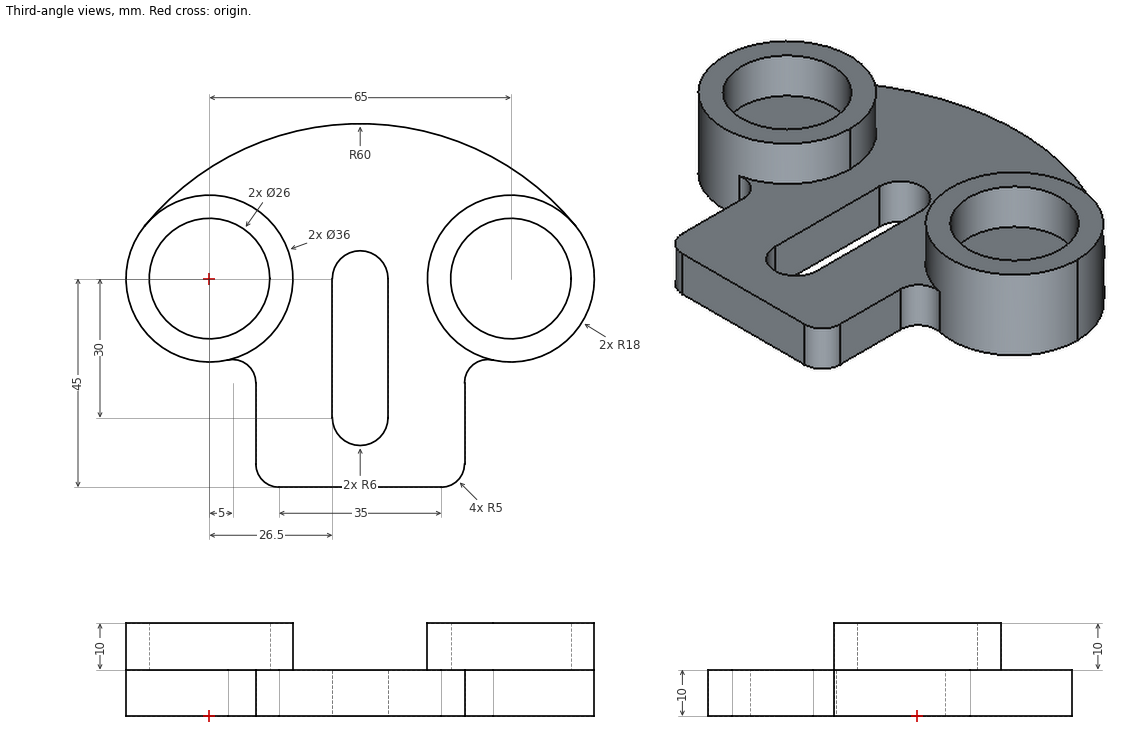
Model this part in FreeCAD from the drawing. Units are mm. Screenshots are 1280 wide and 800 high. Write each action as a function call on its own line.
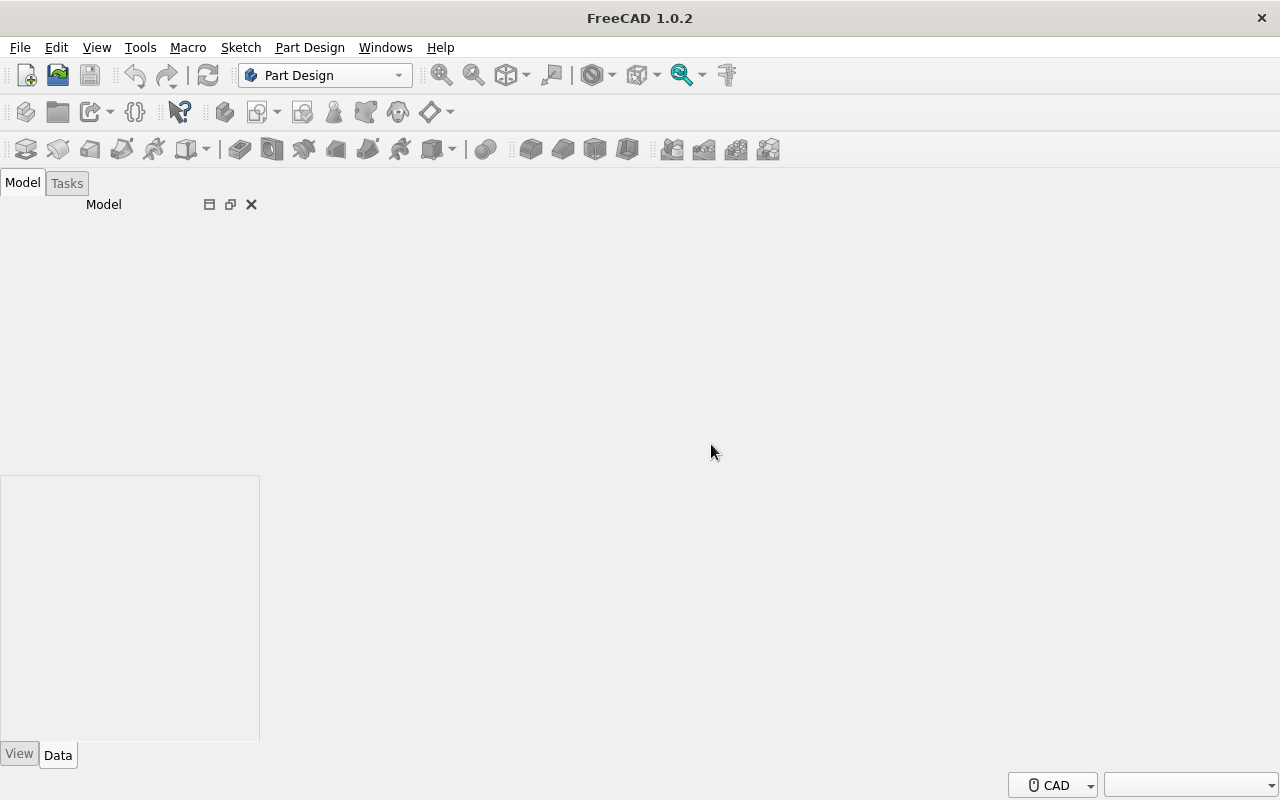
click(26, 76)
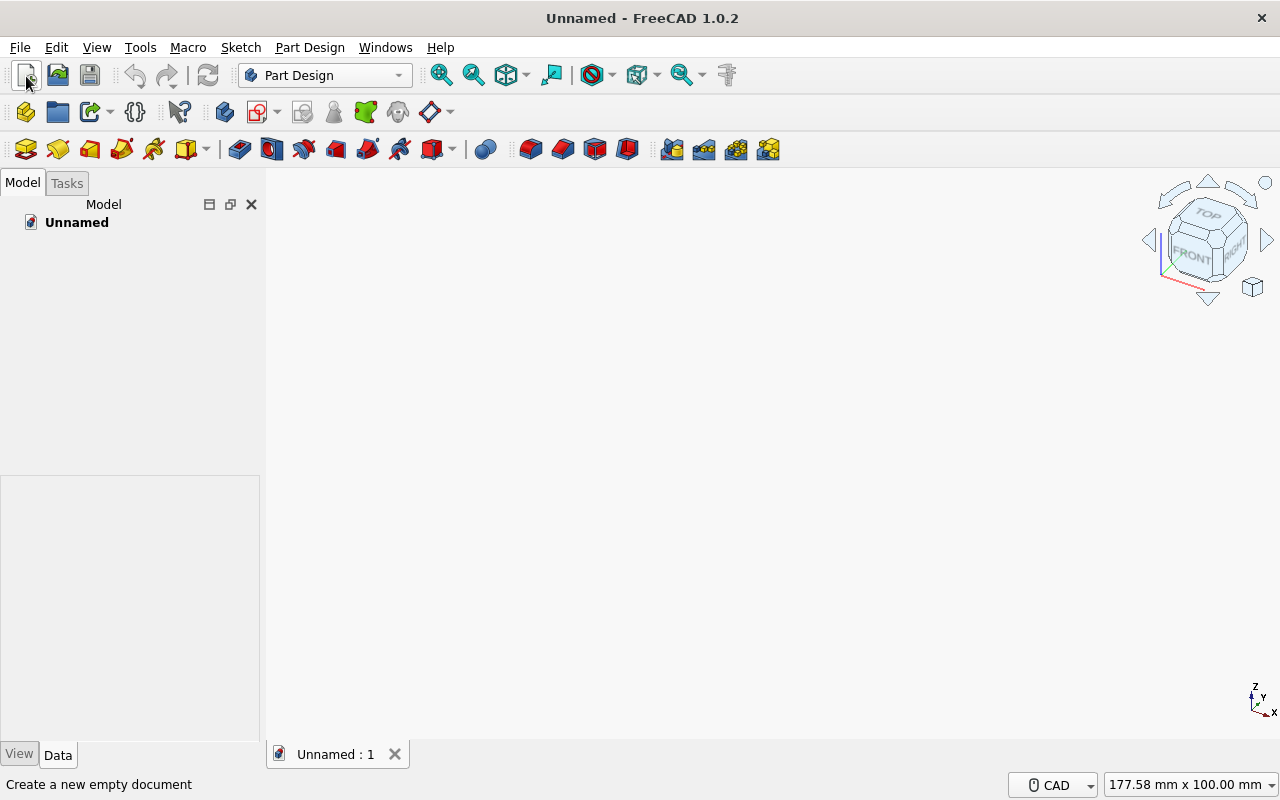
click(258, 112)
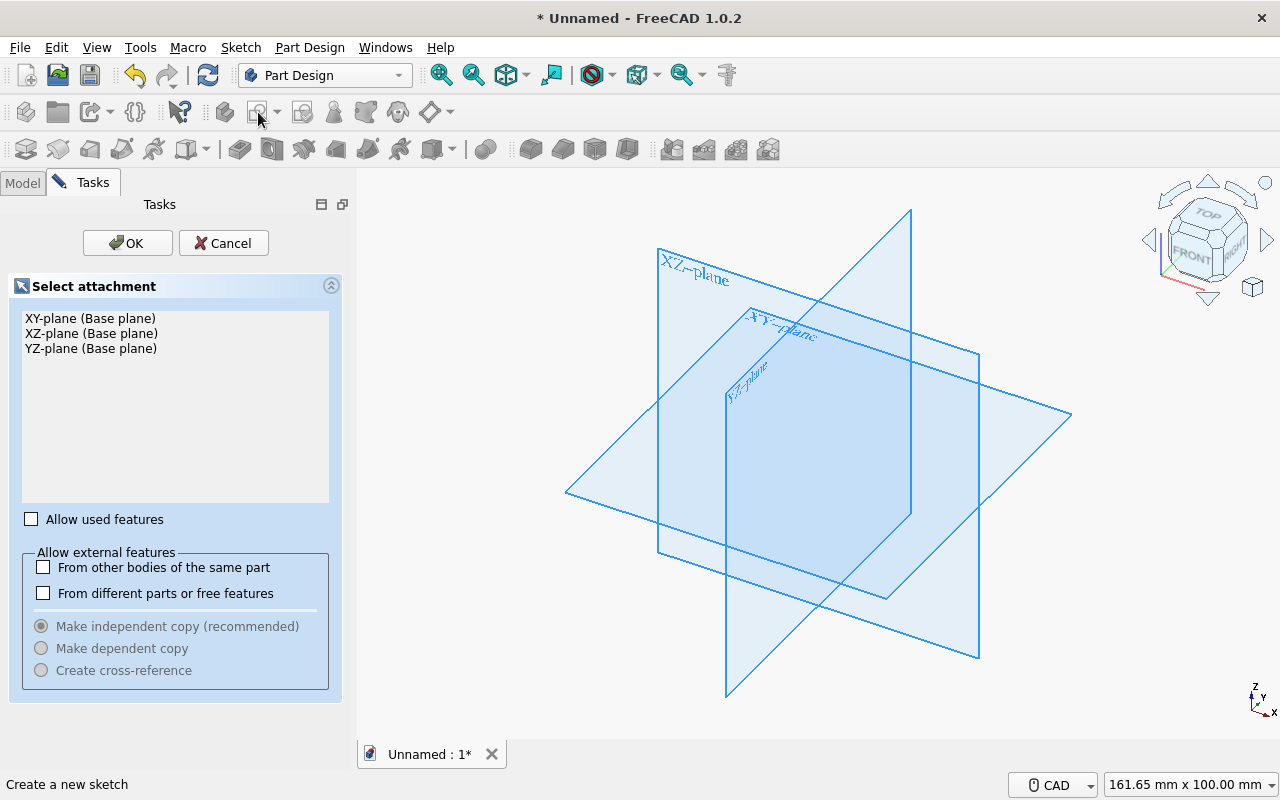
click(82, 318)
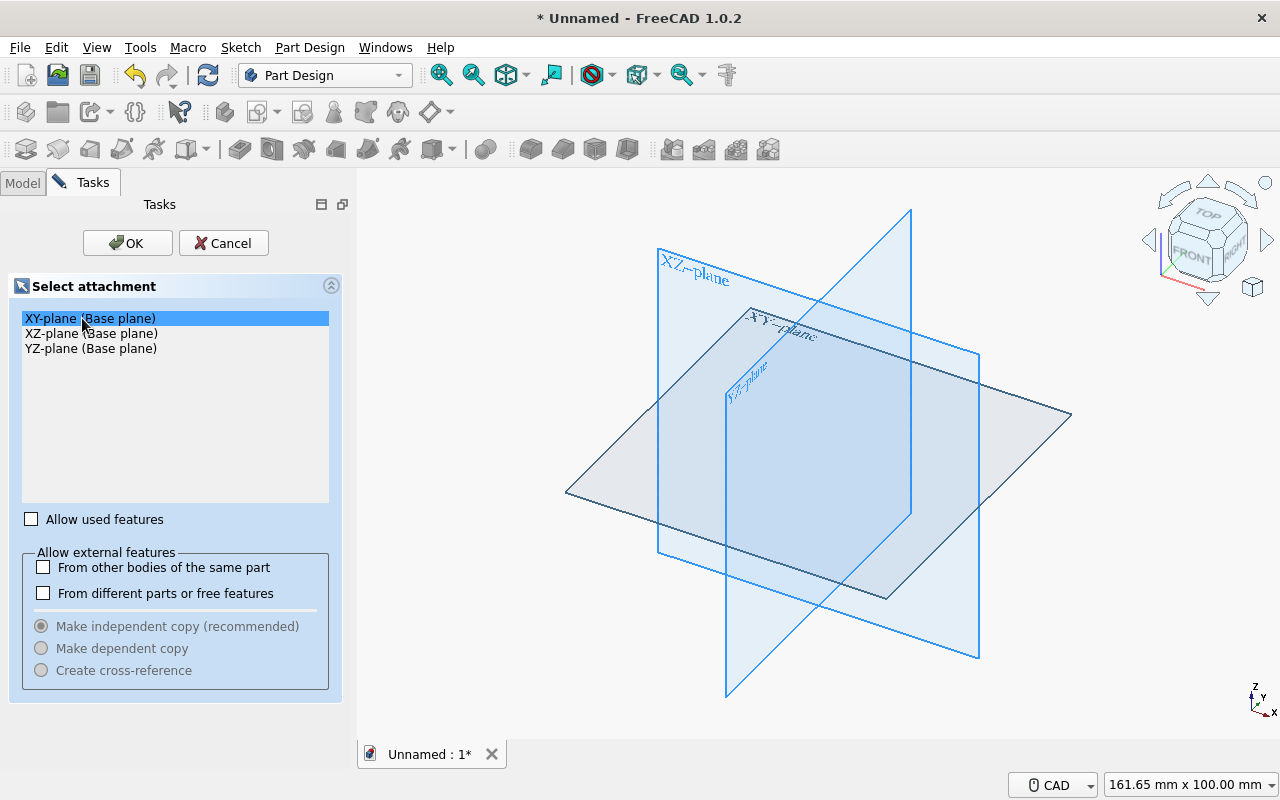
click(128, 243)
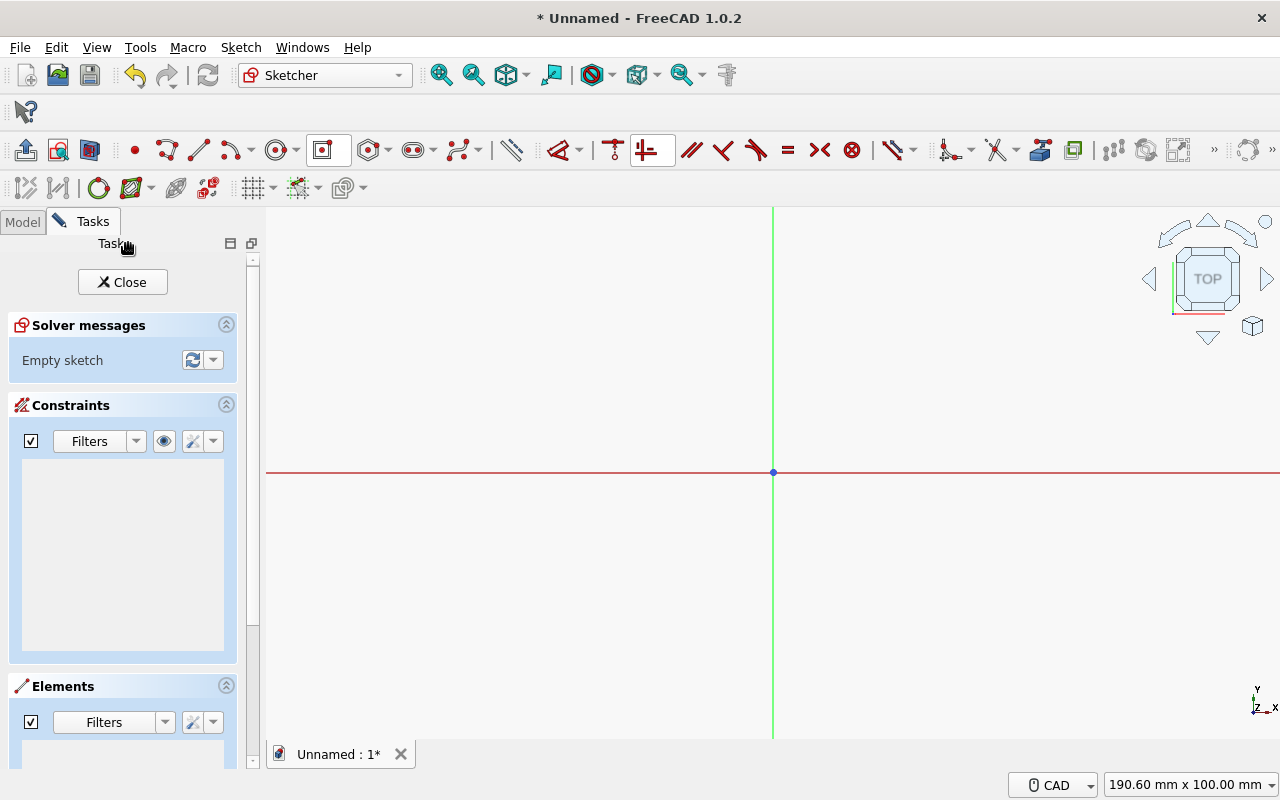
scroll(294, 334, down, 1)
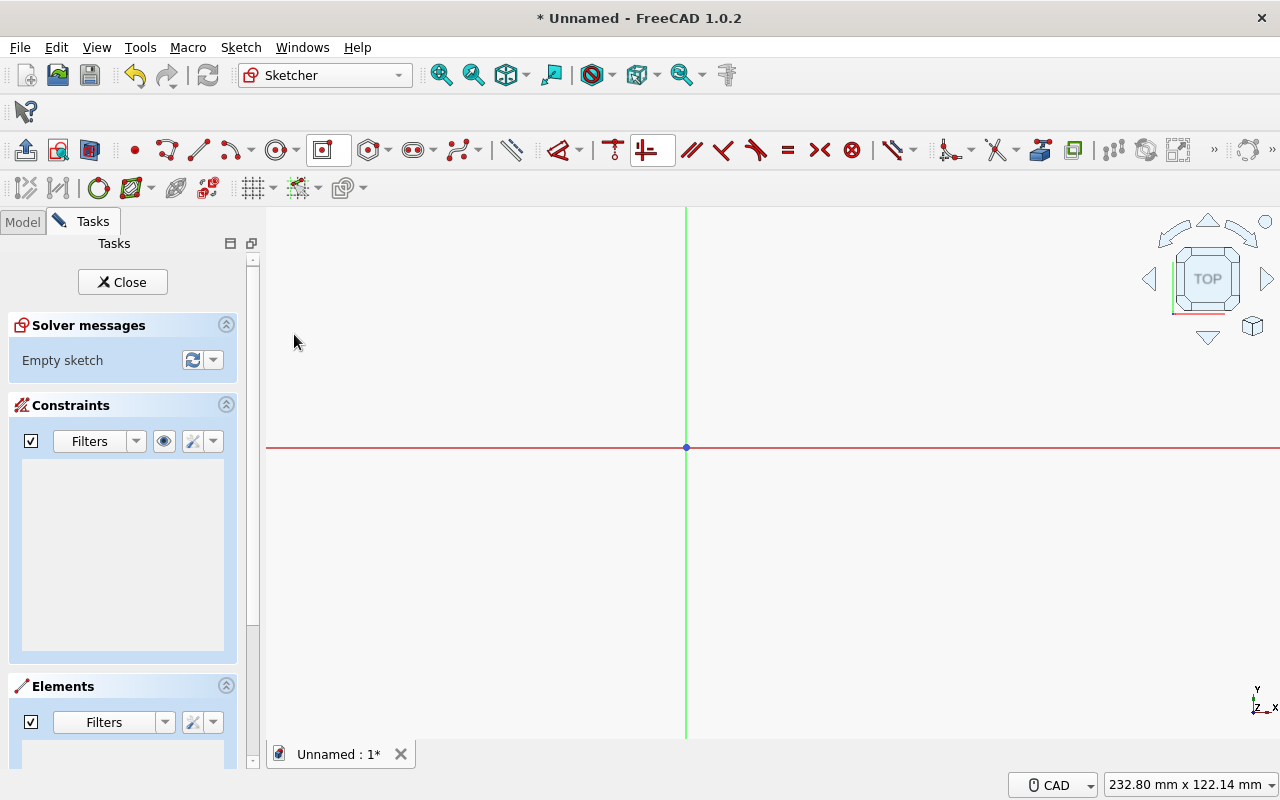
click(200, 150)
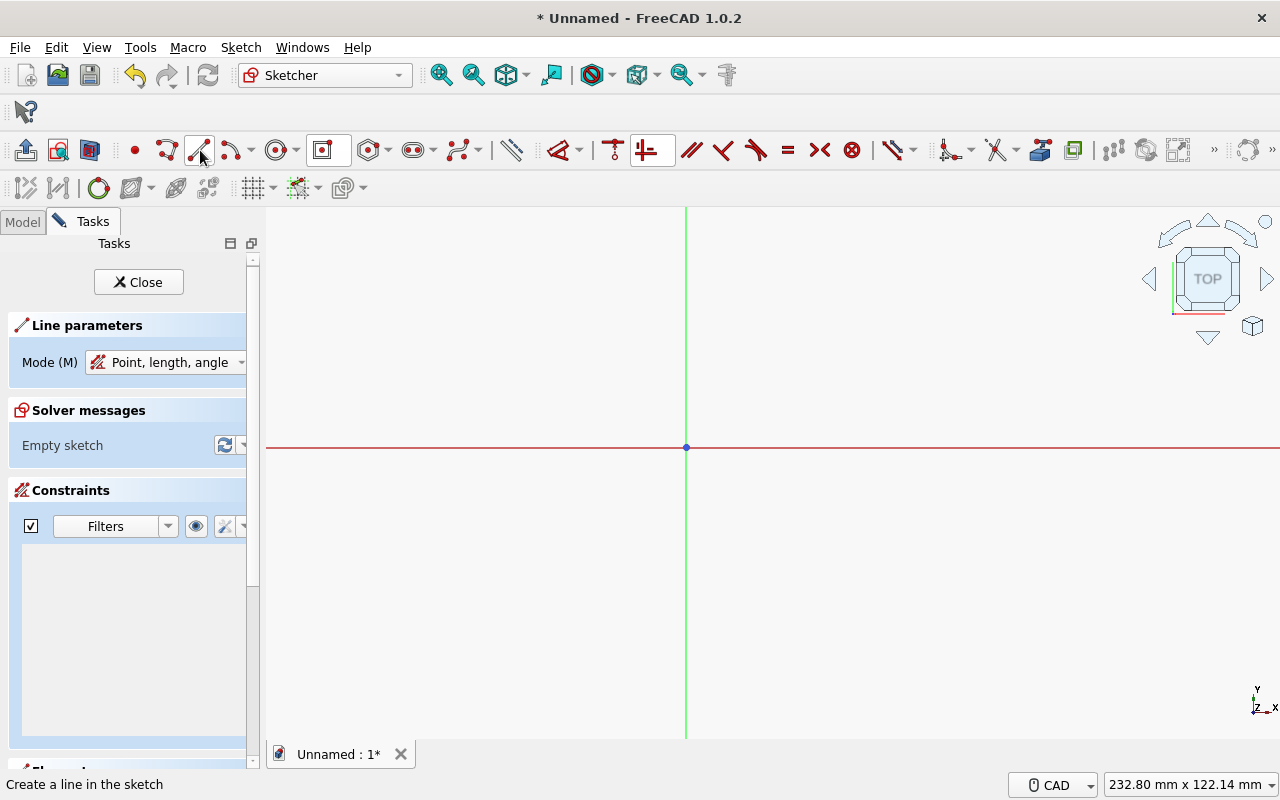
click(752, 644)
click(904, 644)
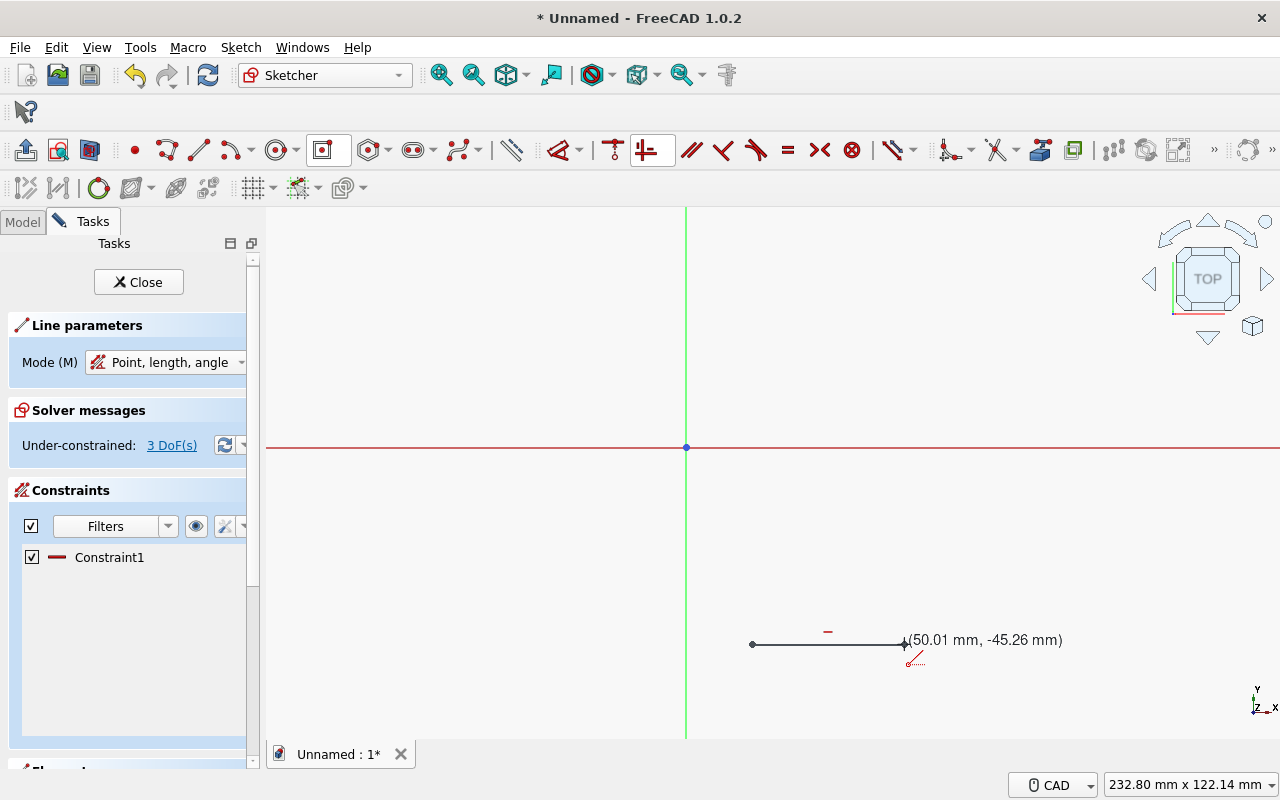
click(926, 622)
click(926, 546)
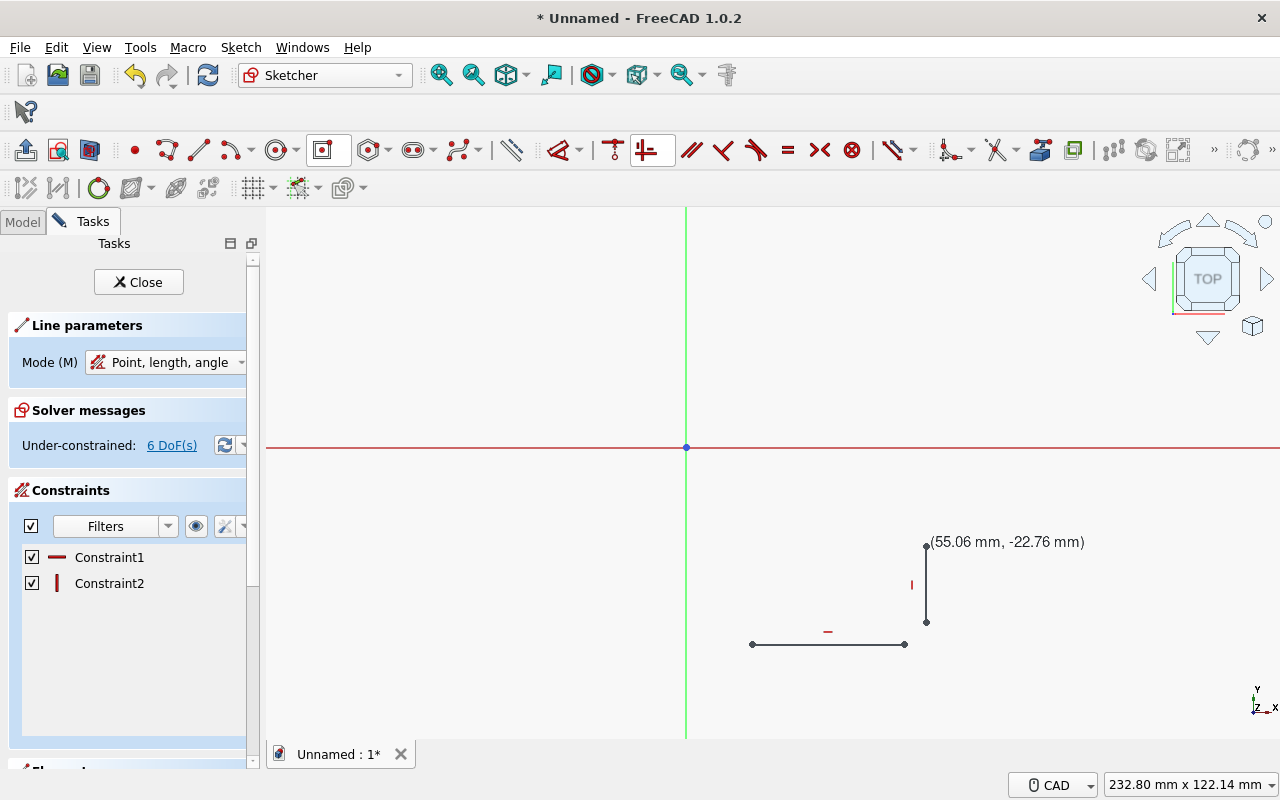
click(730, 546)
click(730, 622)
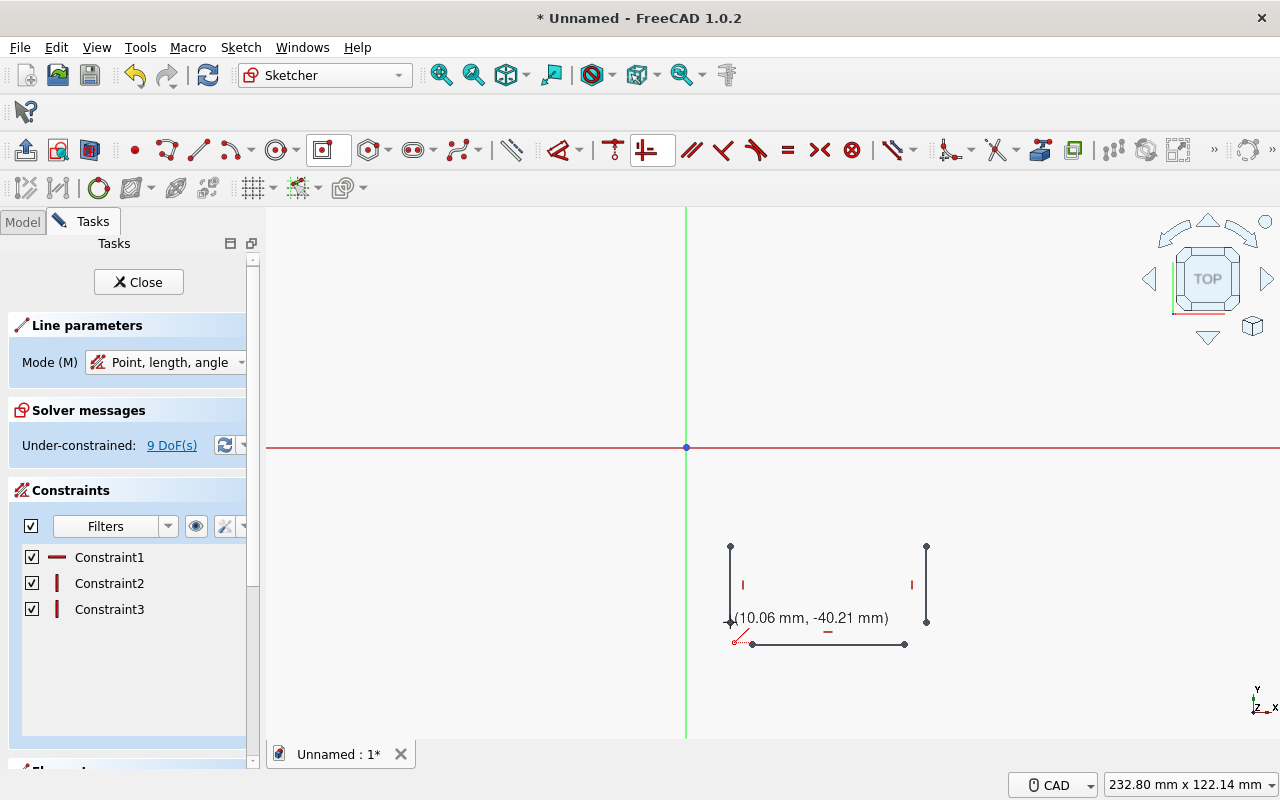
click(254, 150)